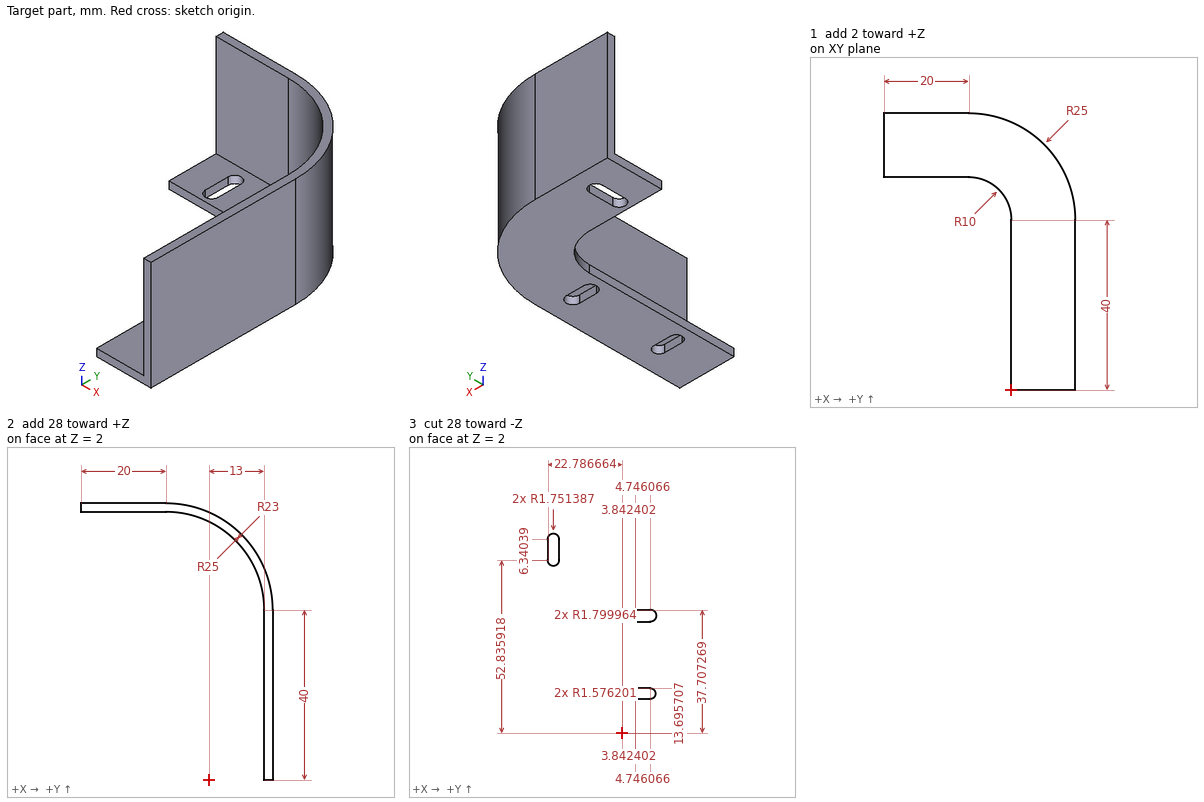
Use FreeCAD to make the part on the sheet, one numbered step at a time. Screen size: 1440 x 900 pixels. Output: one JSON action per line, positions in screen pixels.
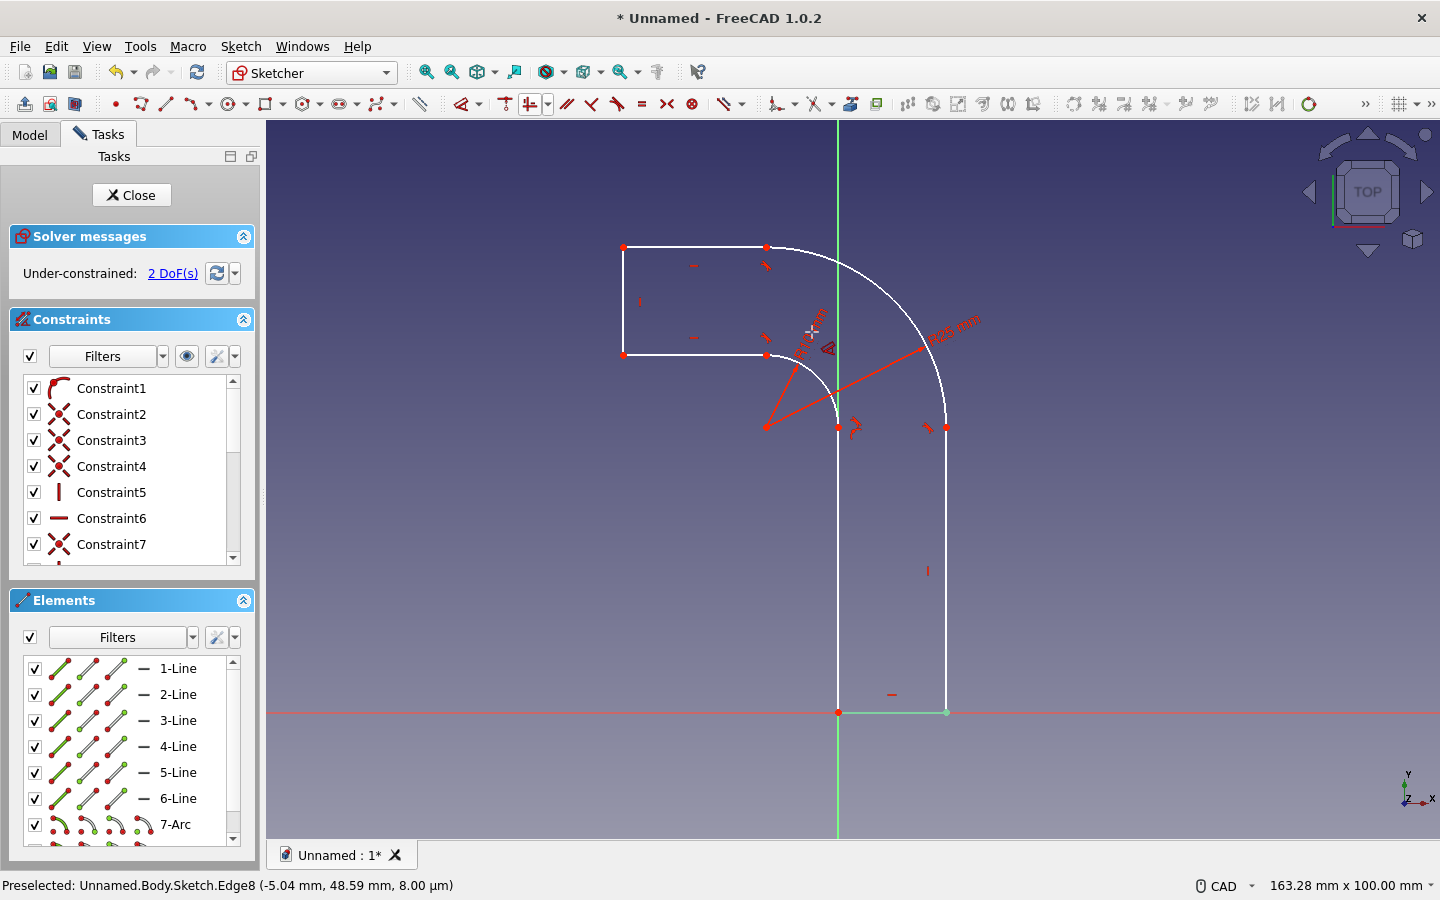
{"action": "left_click", "coordinate": [838, 513]}
{"action": "left_click", "coordinate": [872, 570]}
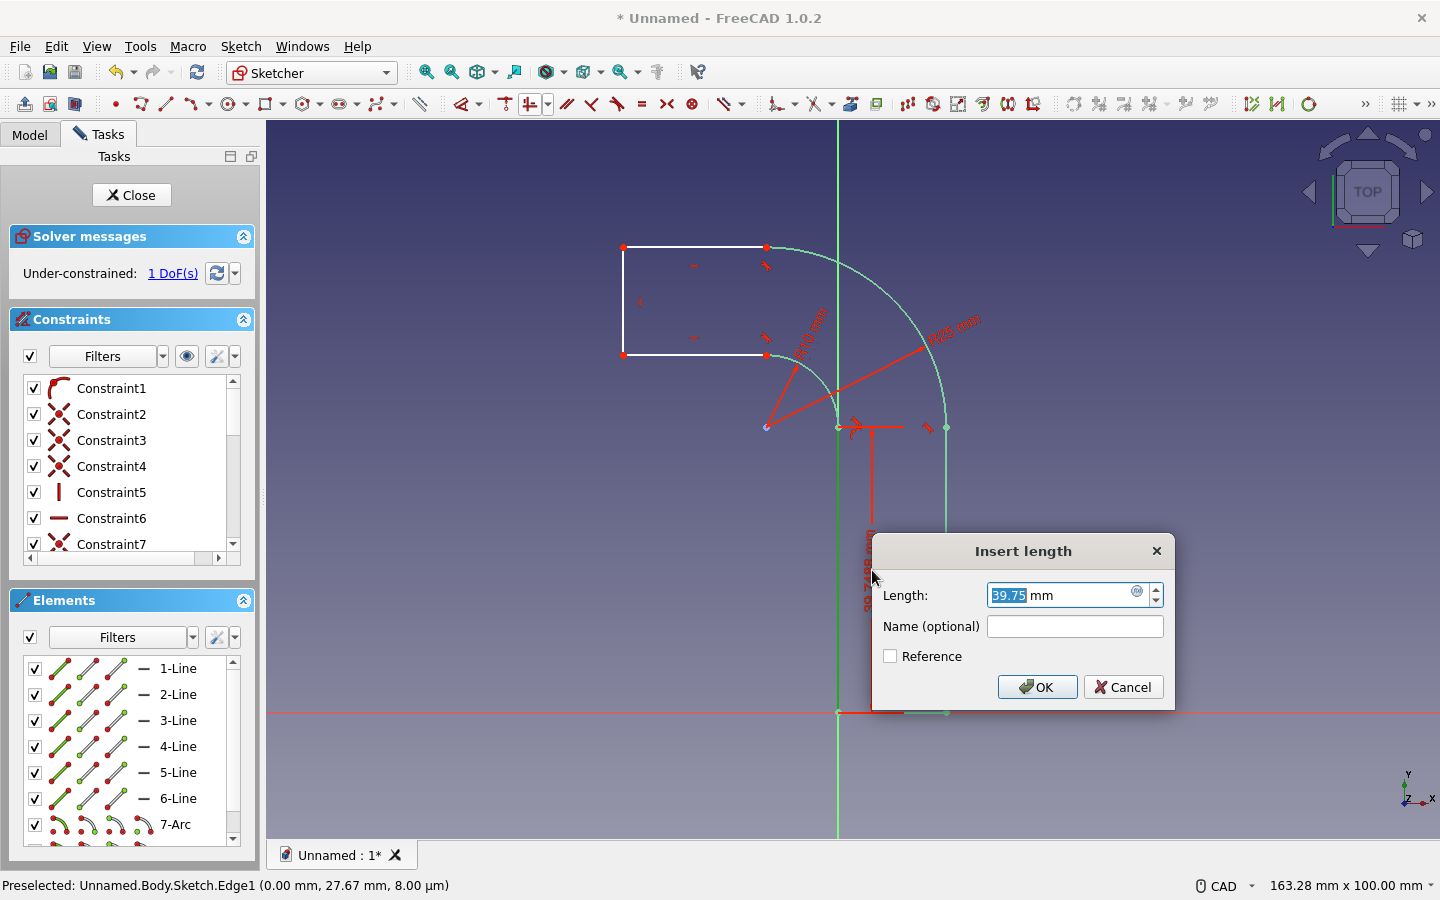
{"action": "type", "text": "40"}
{"action": "key", "text": "Return"}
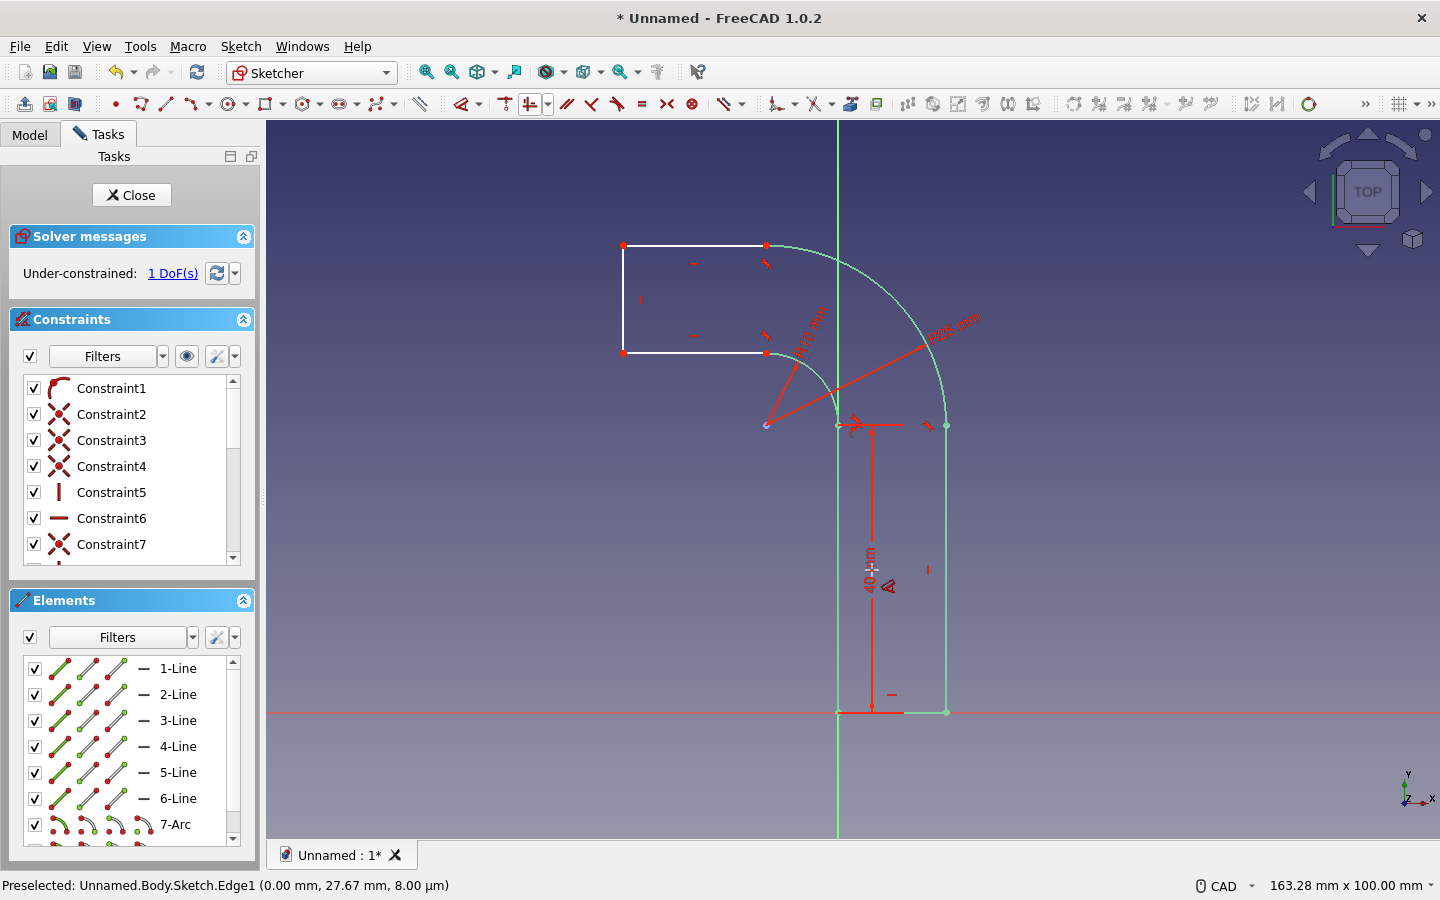
{"action": "left_click", "coordinate": [723, 246]}
{"action": "left_click", "coordinate": [695, 212]}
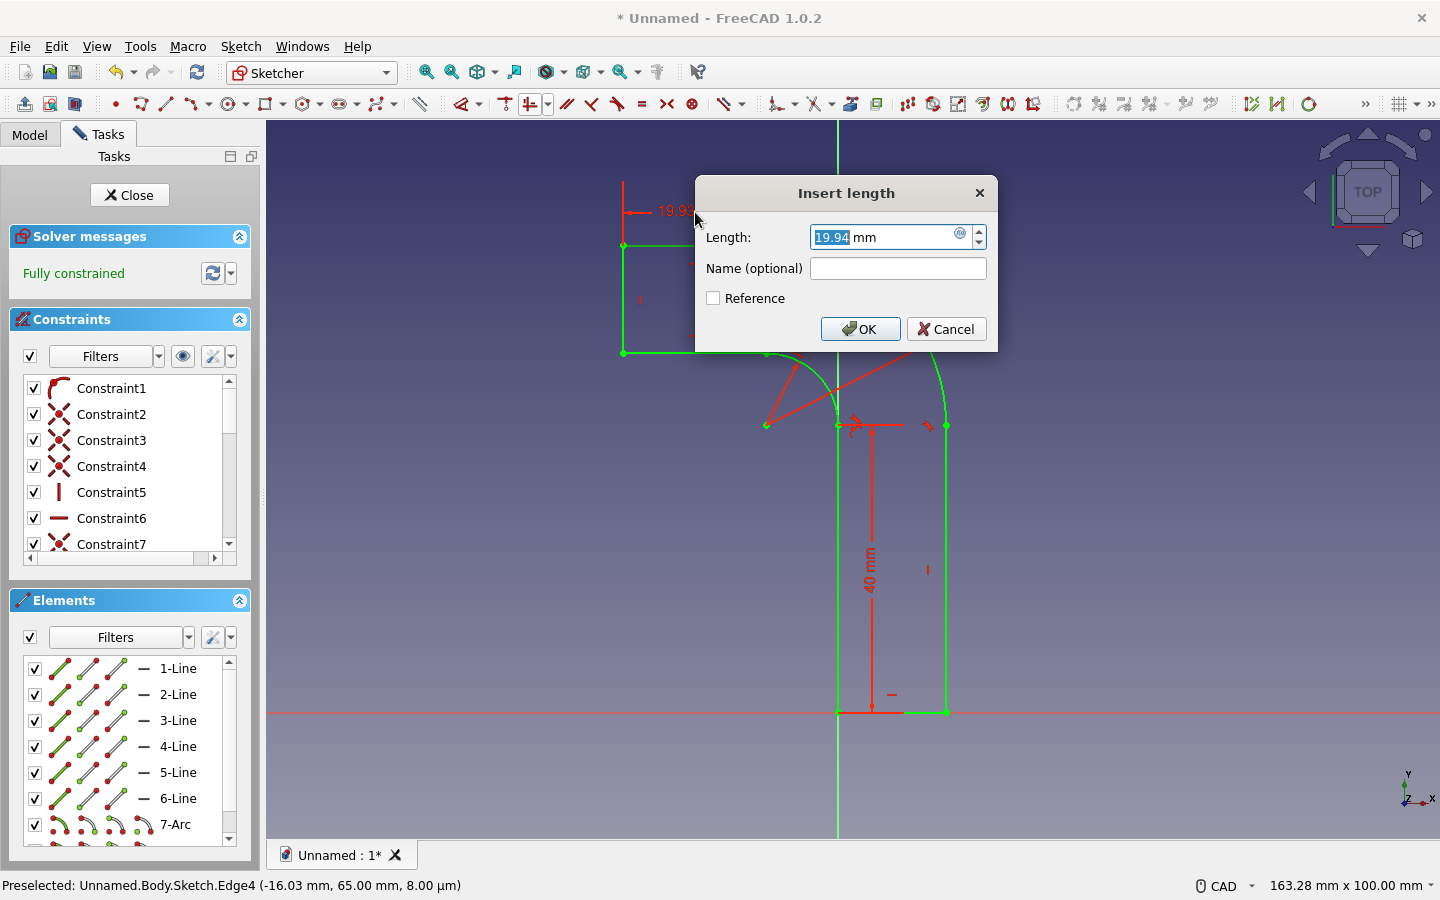
{"action": "type", "text": "20"}
{"action": "key", "text": "Return"}
{"action": "key", "text": "Escape"}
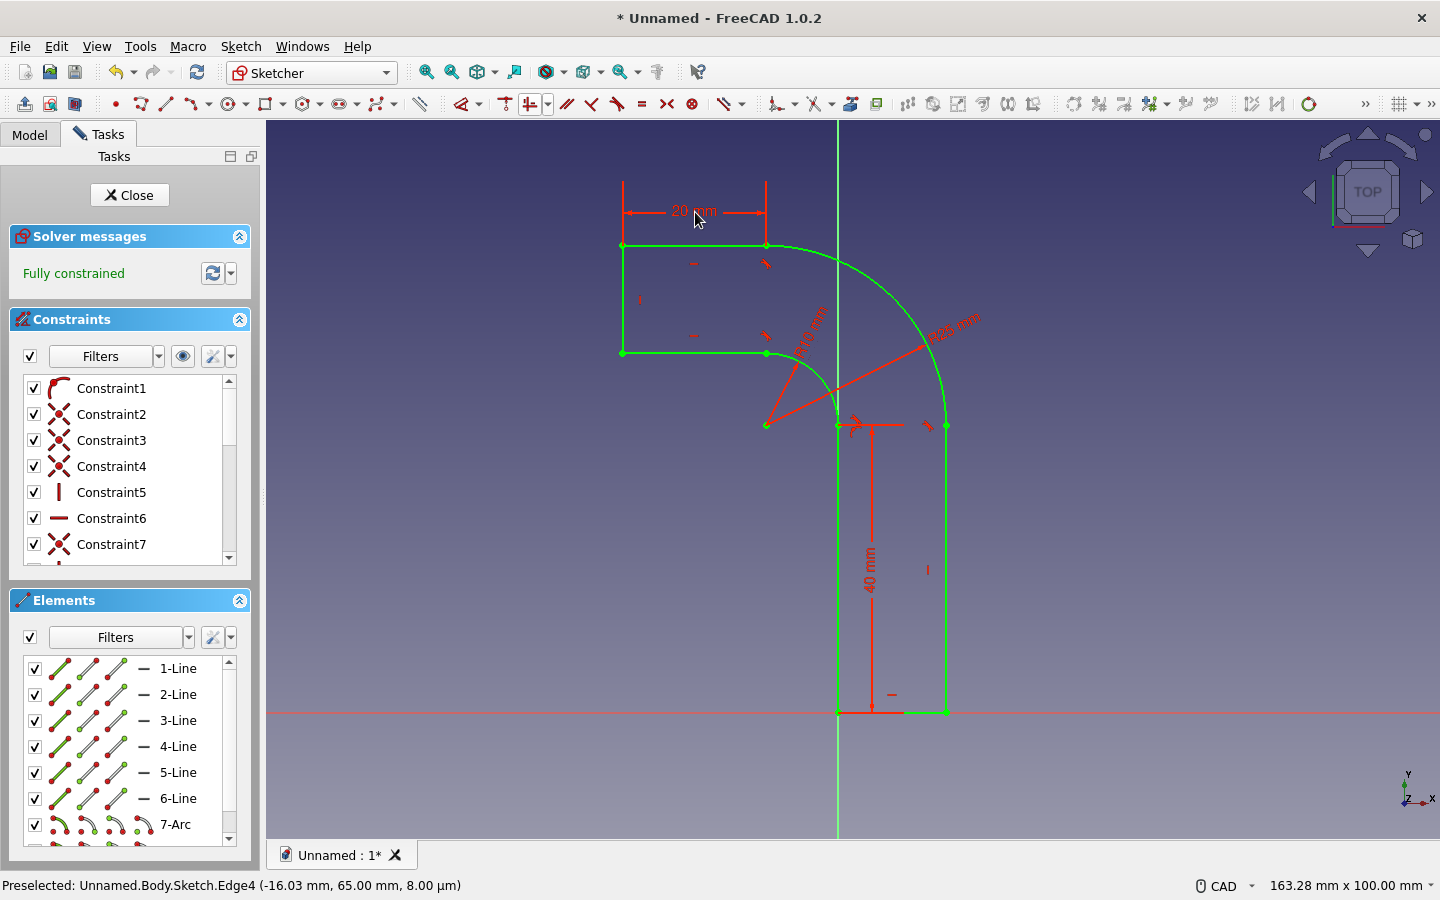
{"action": "left_click", "coordinate": [130, 195]}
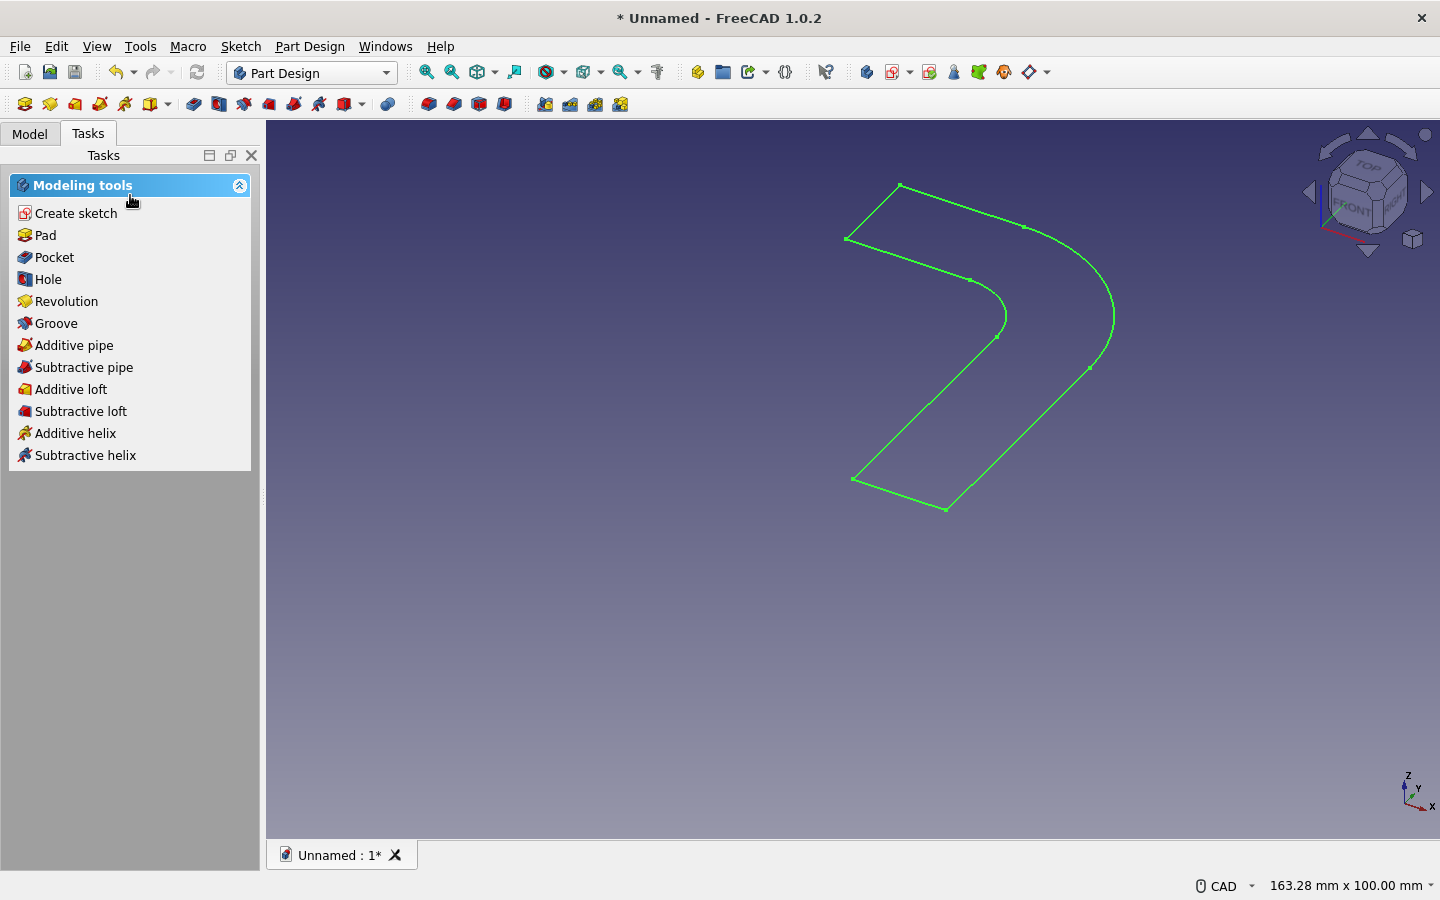
{"action": "left_click", "coordinate": [25, 104]}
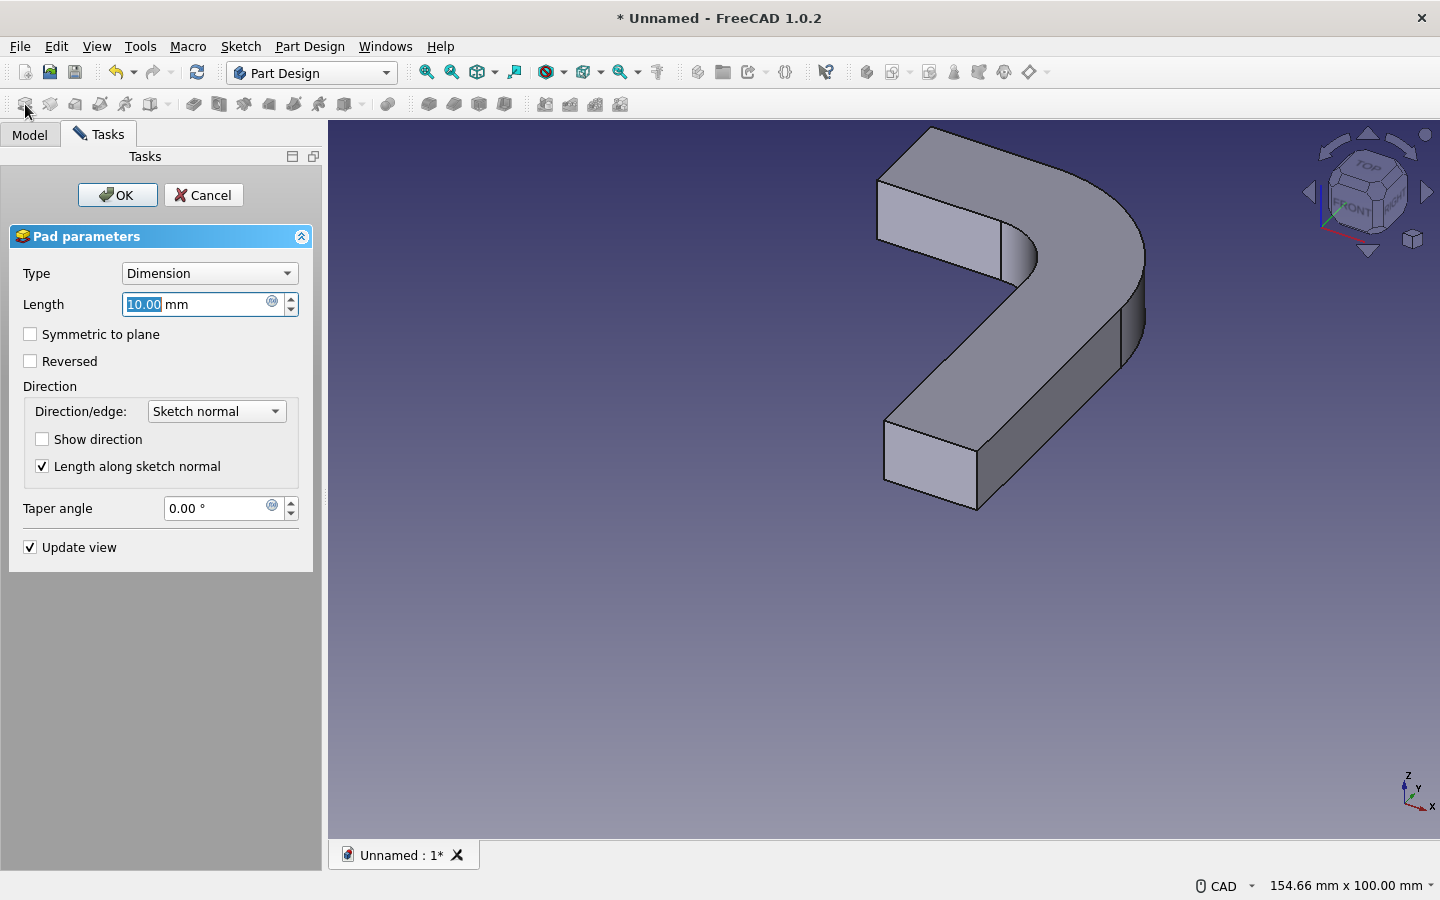
{"action": "type", "text": "2"}
{"action": "key", "text": "Tab"}